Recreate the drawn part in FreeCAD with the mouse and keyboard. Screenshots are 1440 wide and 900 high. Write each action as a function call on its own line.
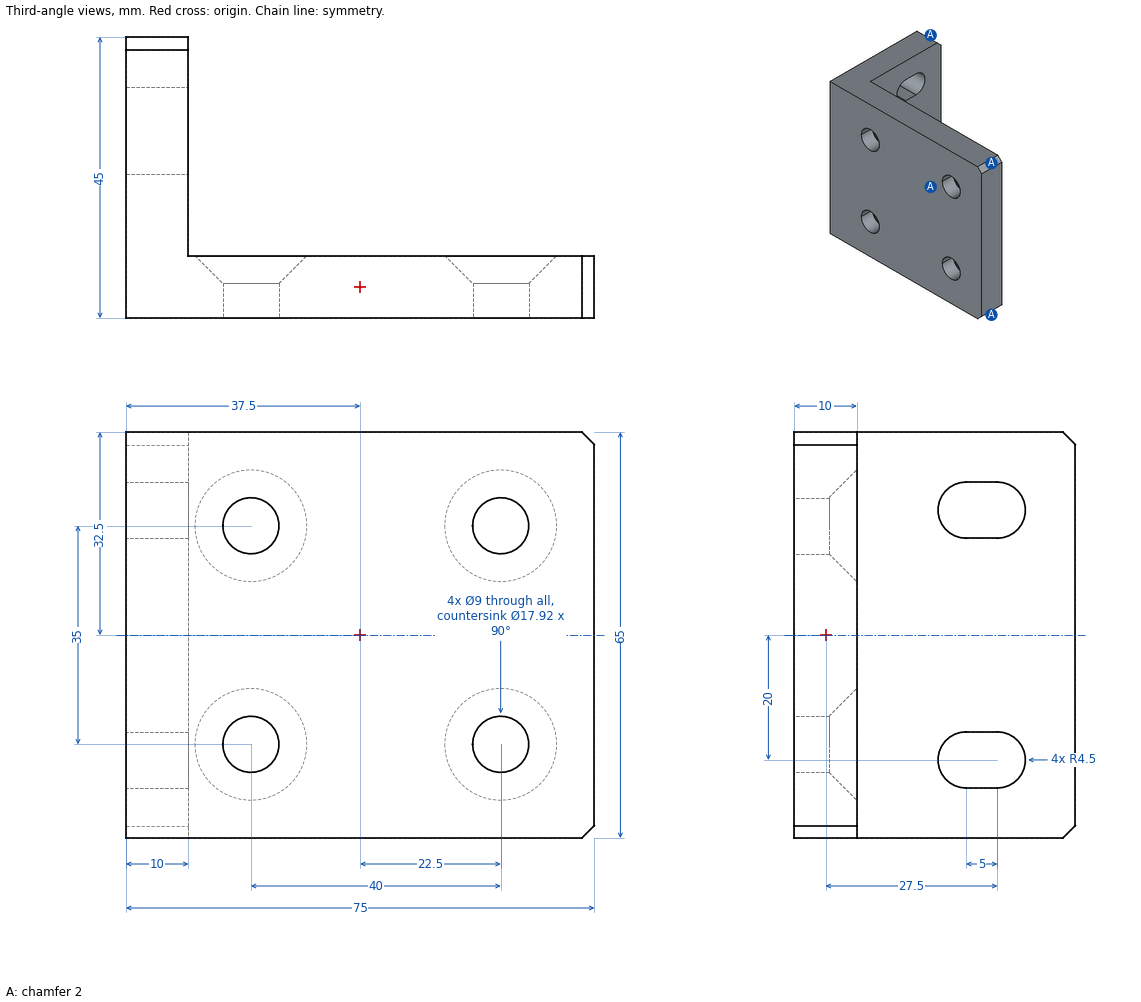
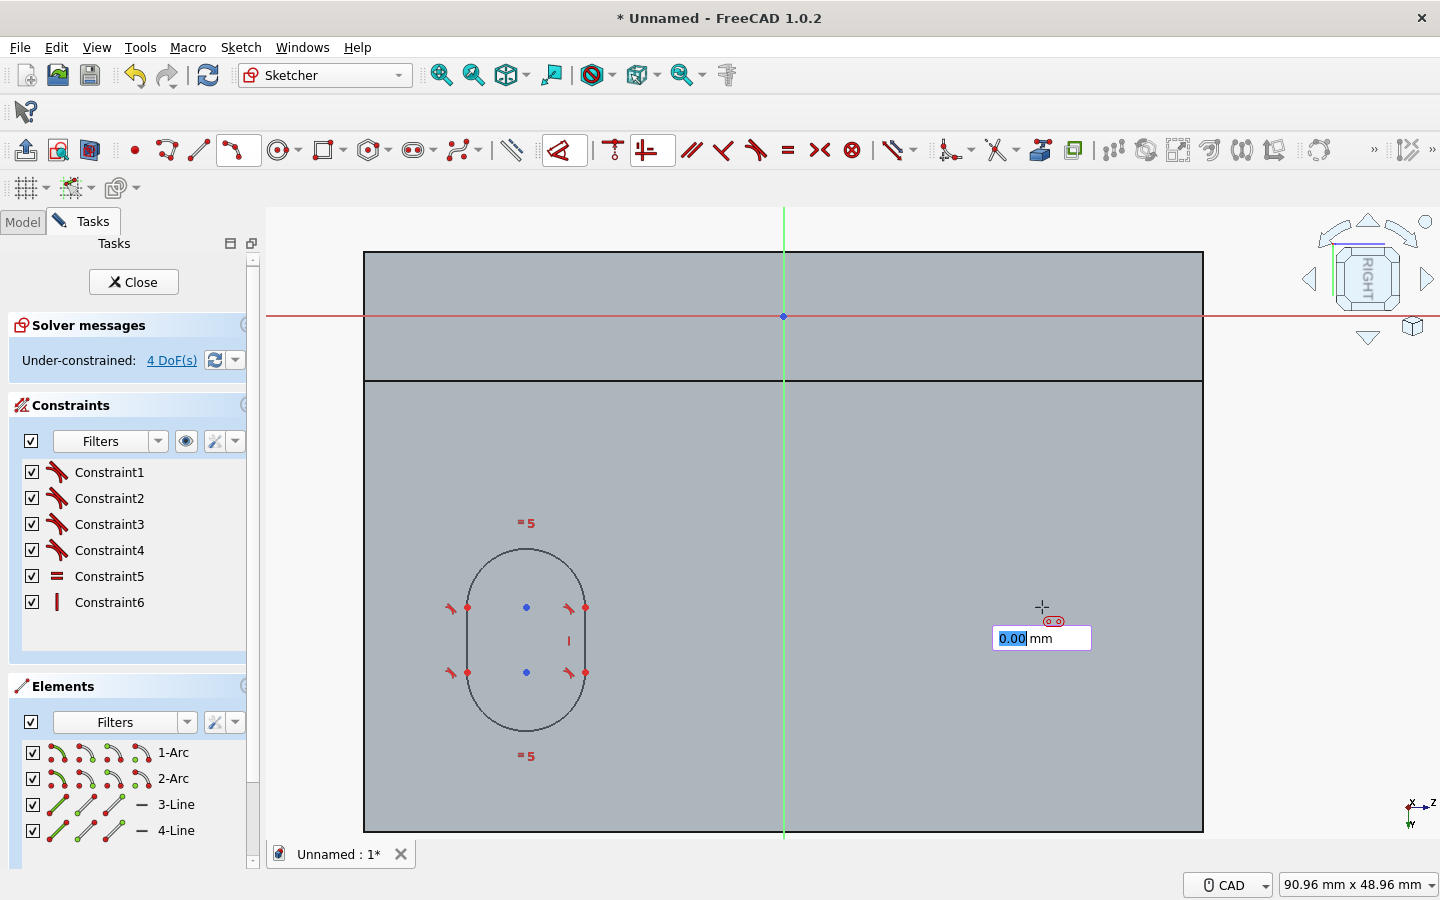
click(1100, 639)
key(Escape)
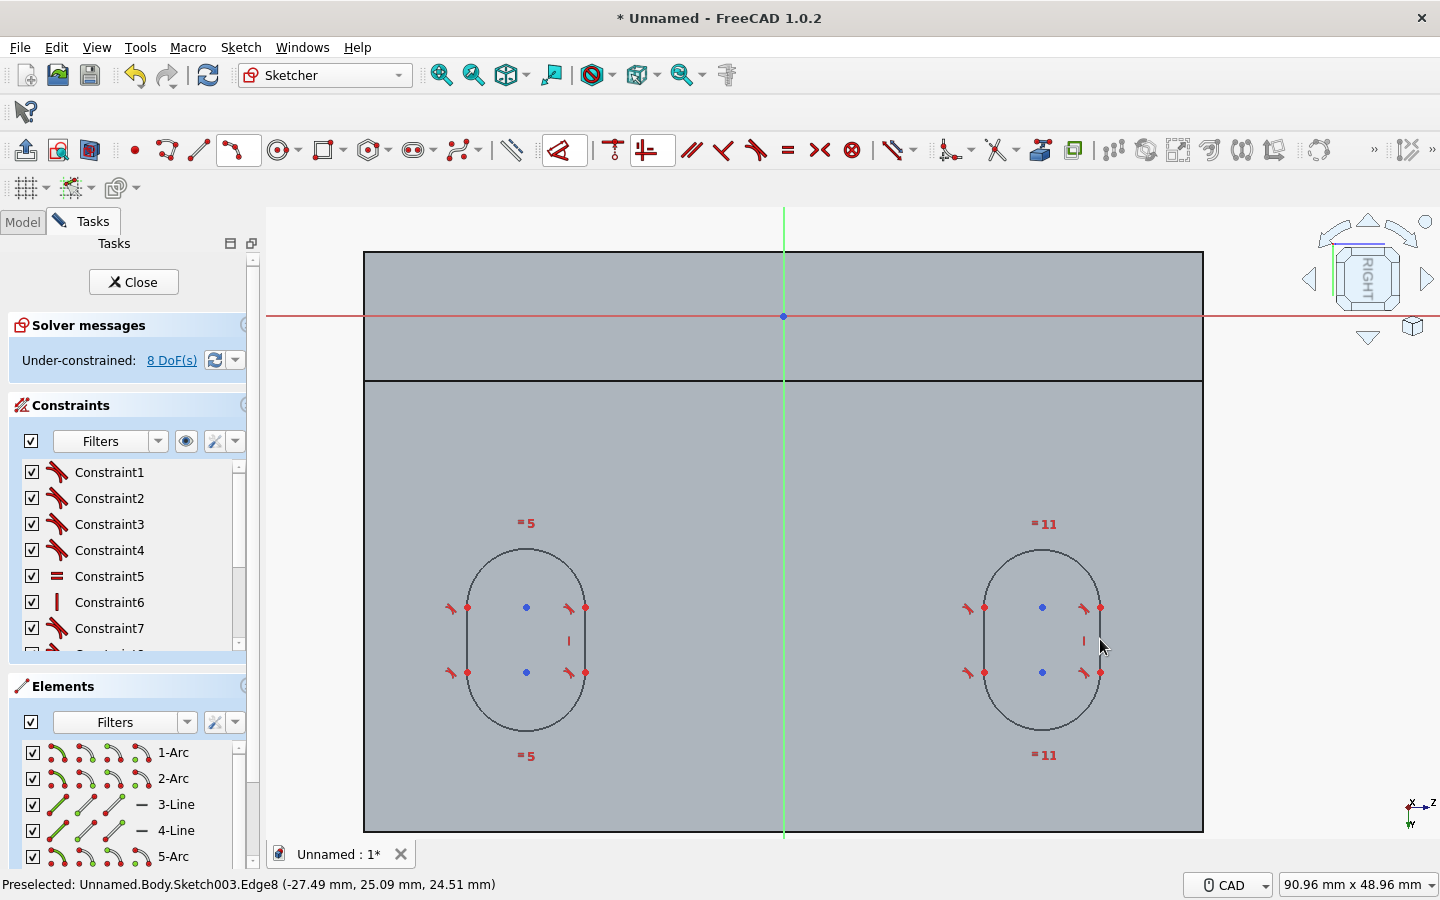
click(491, 720)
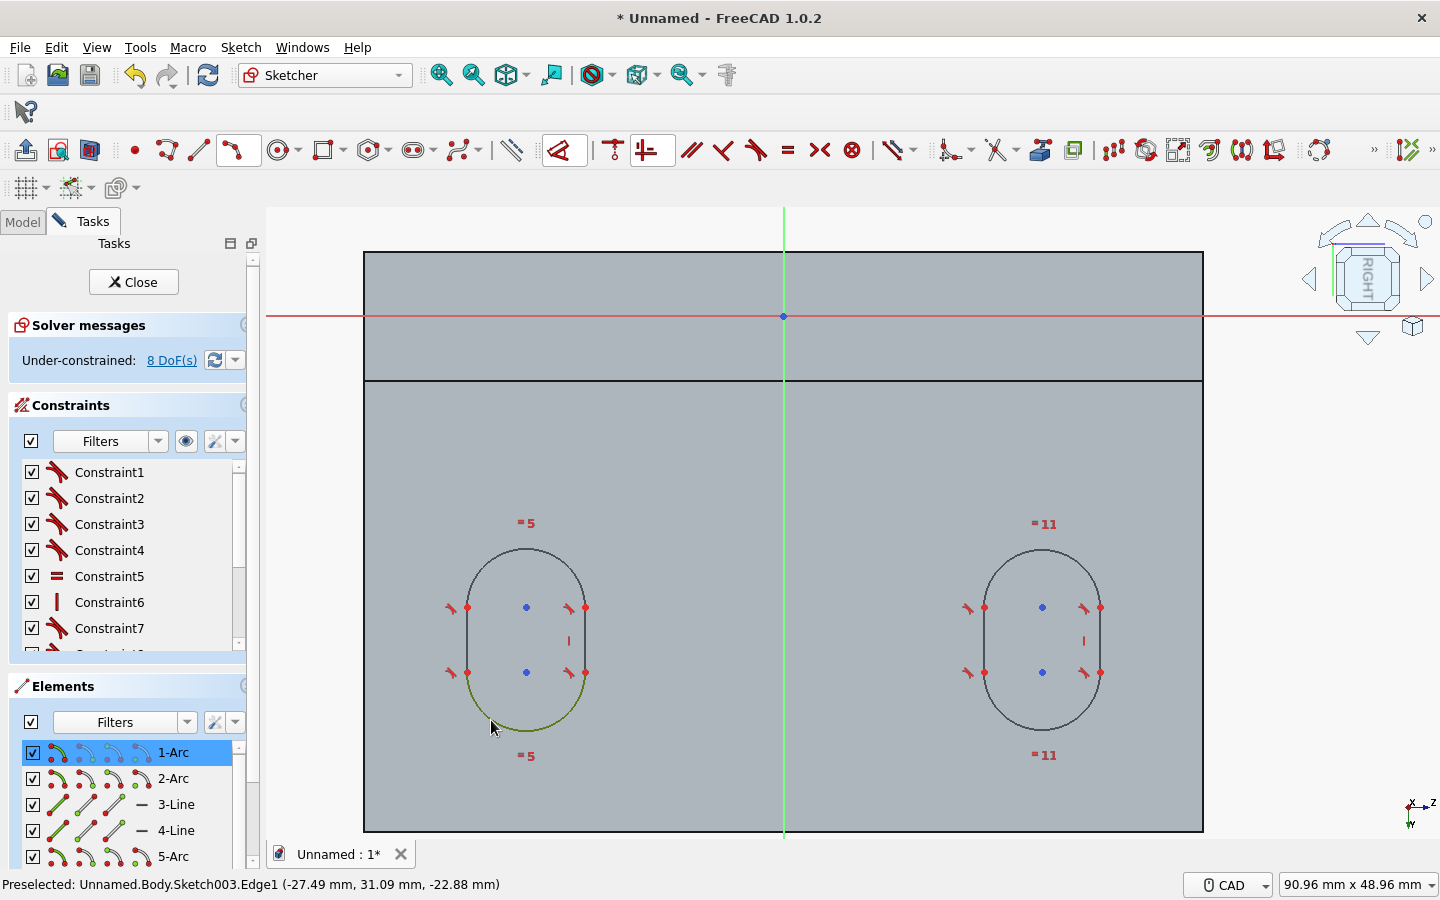
click(1008, 719)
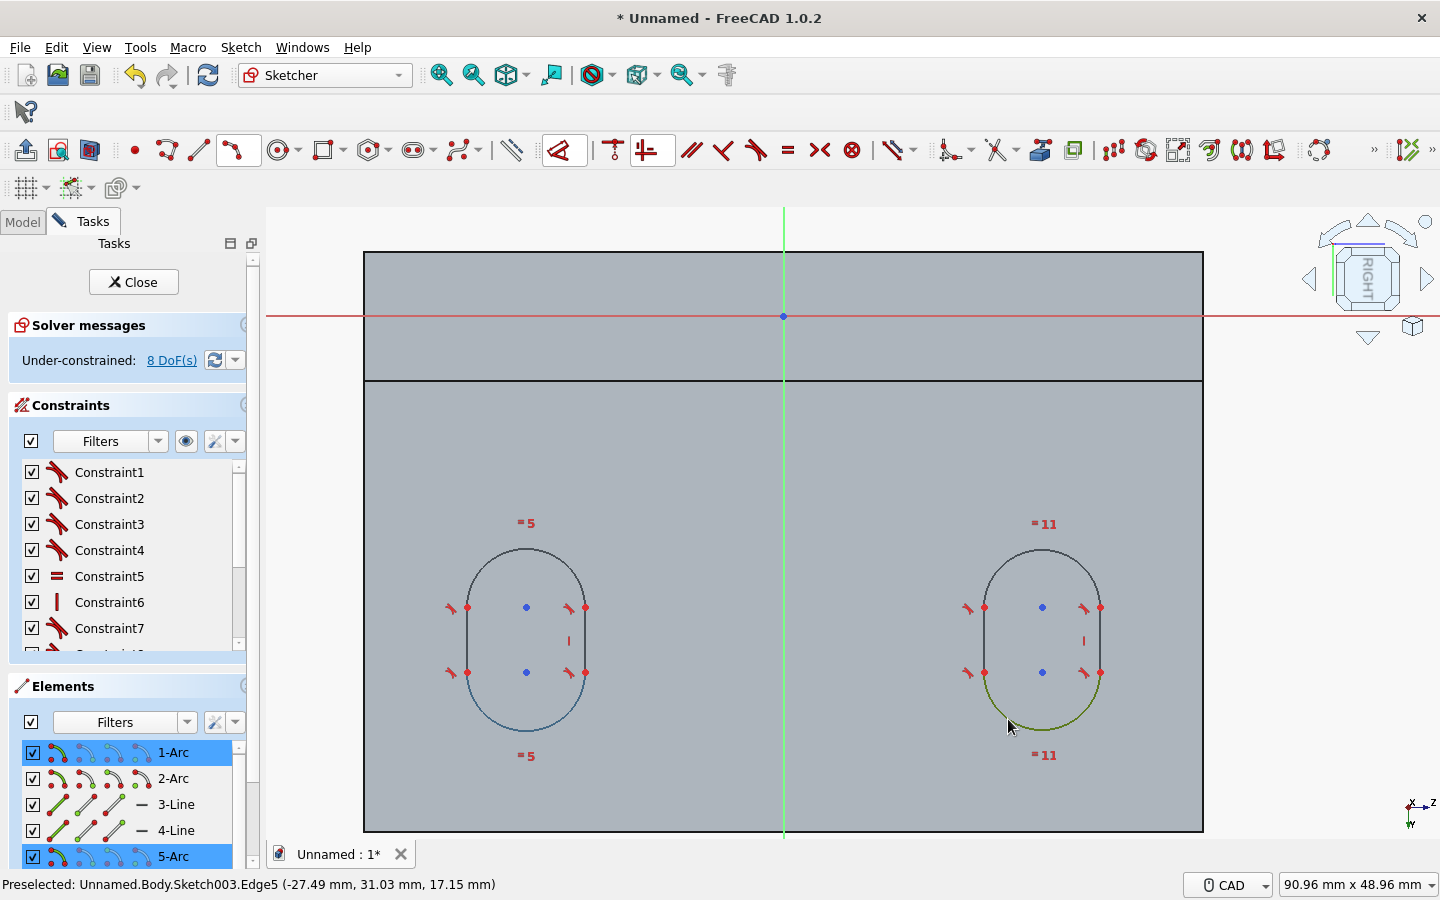
key(e)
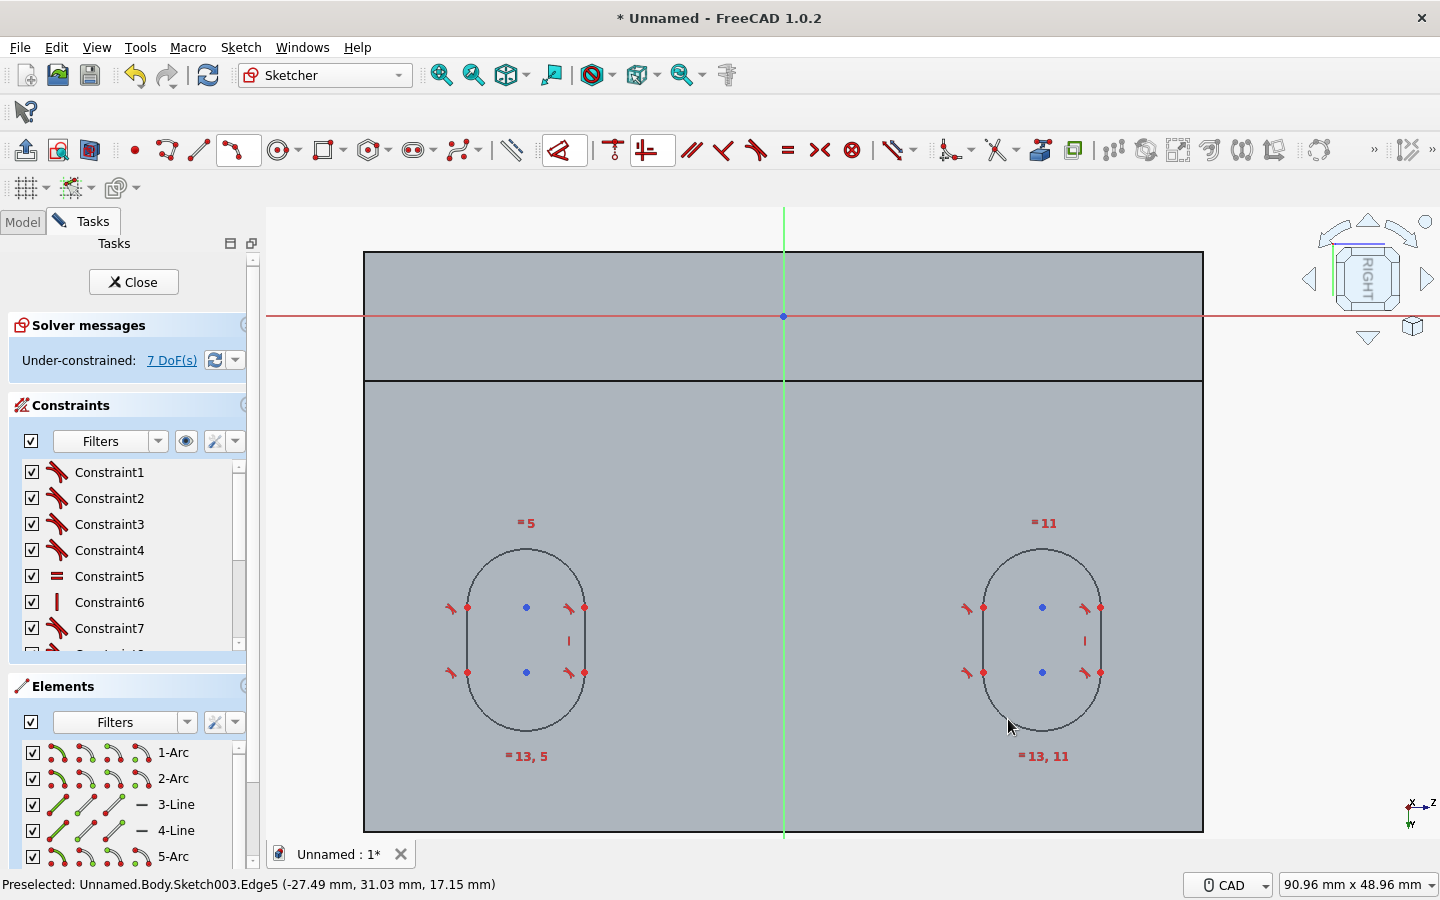
click(526, 672)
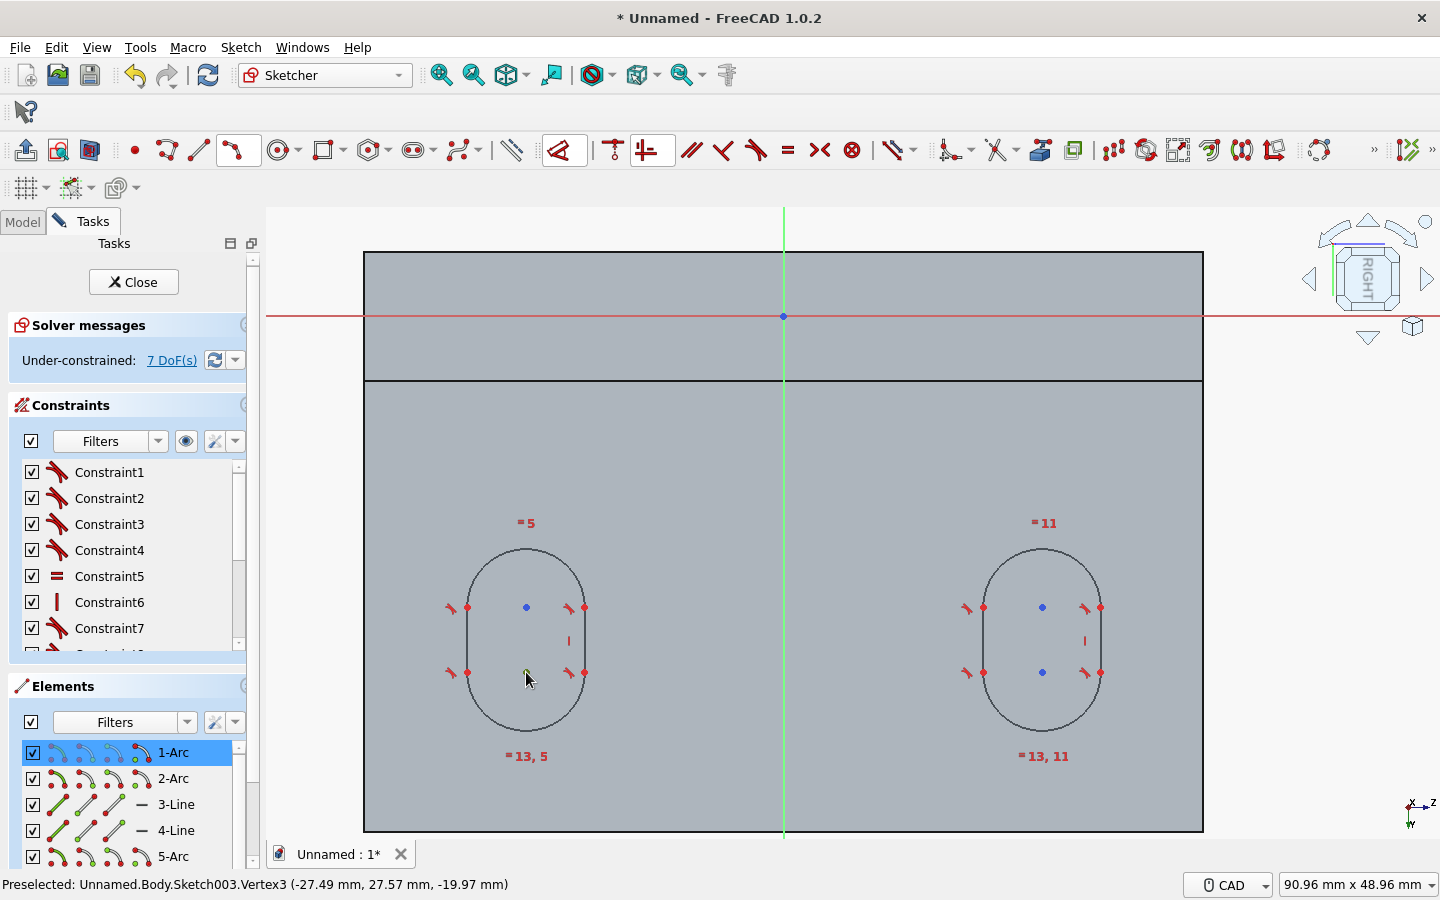
click(1042, 672)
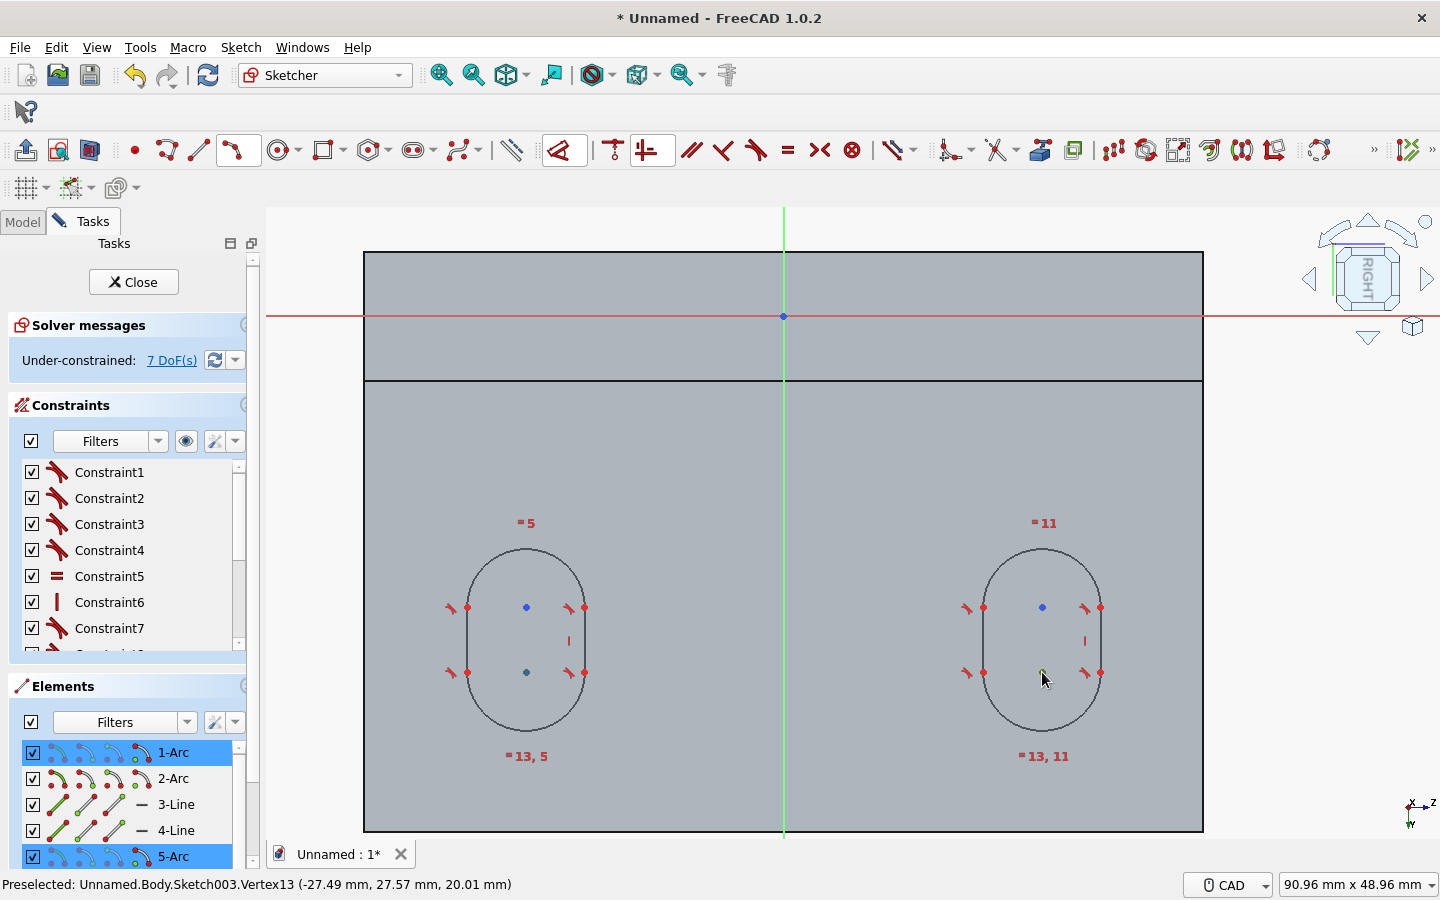
click(784, 770)